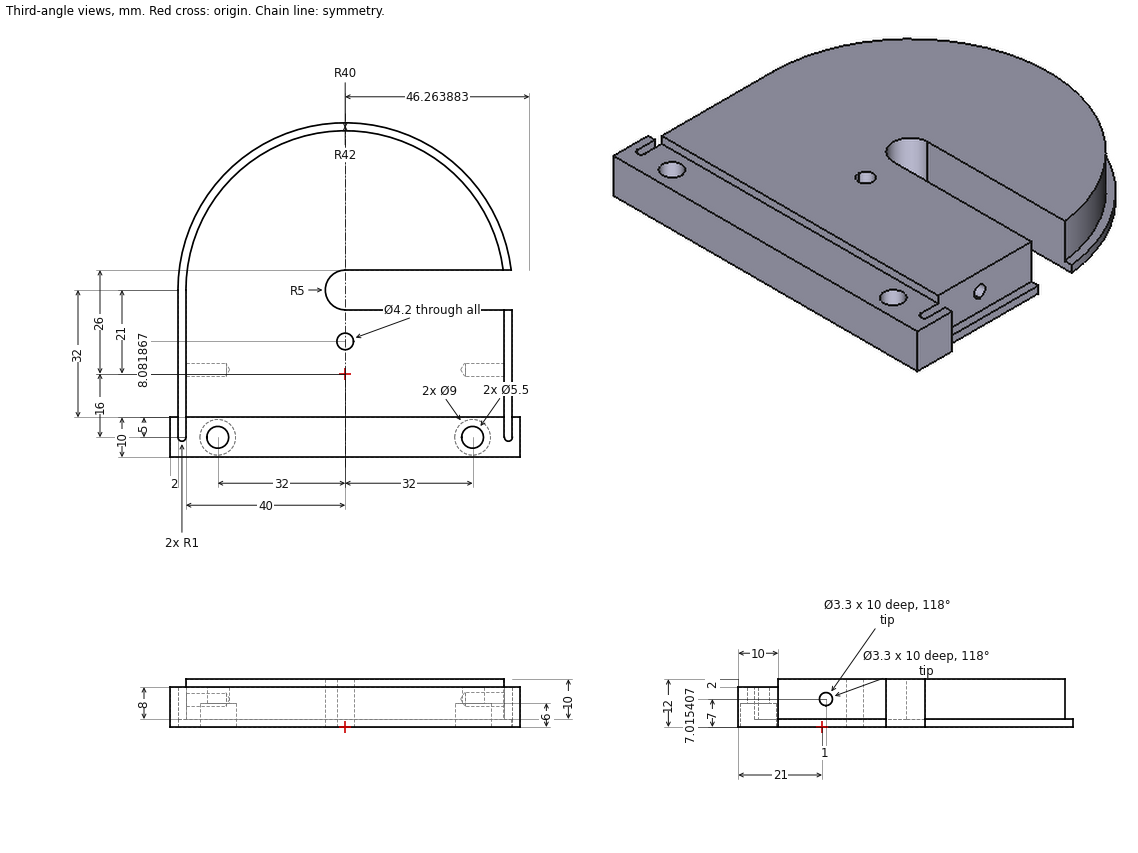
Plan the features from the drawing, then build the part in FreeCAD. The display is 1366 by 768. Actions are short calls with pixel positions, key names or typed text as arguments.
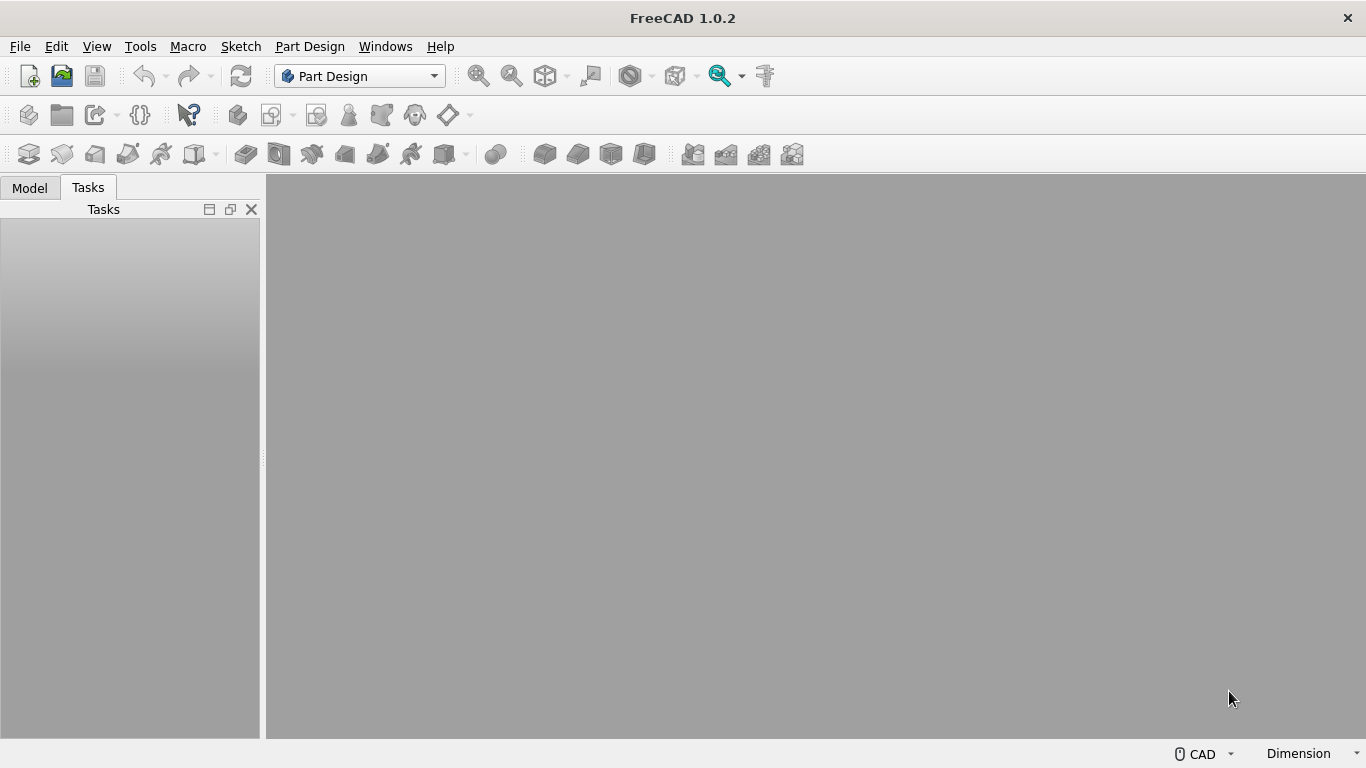
click(29, 76)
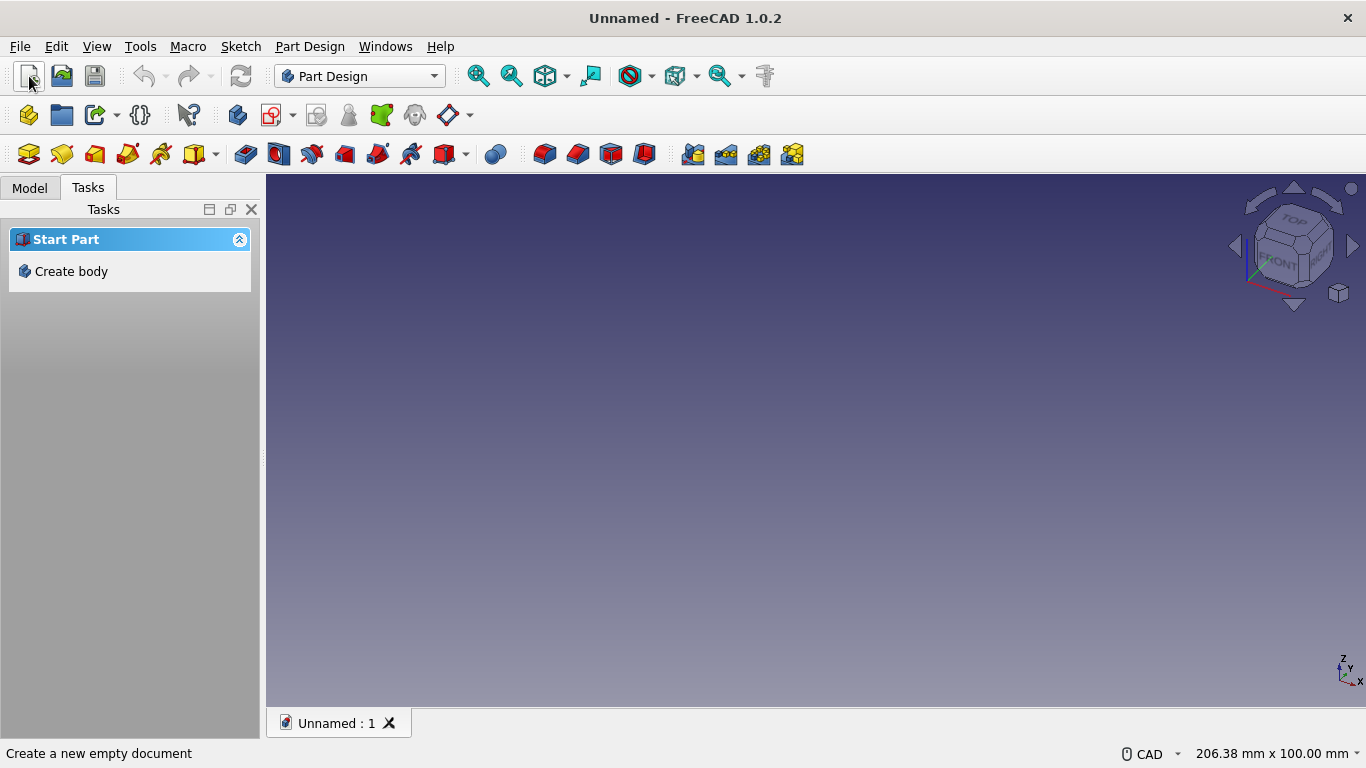
click(270, 116)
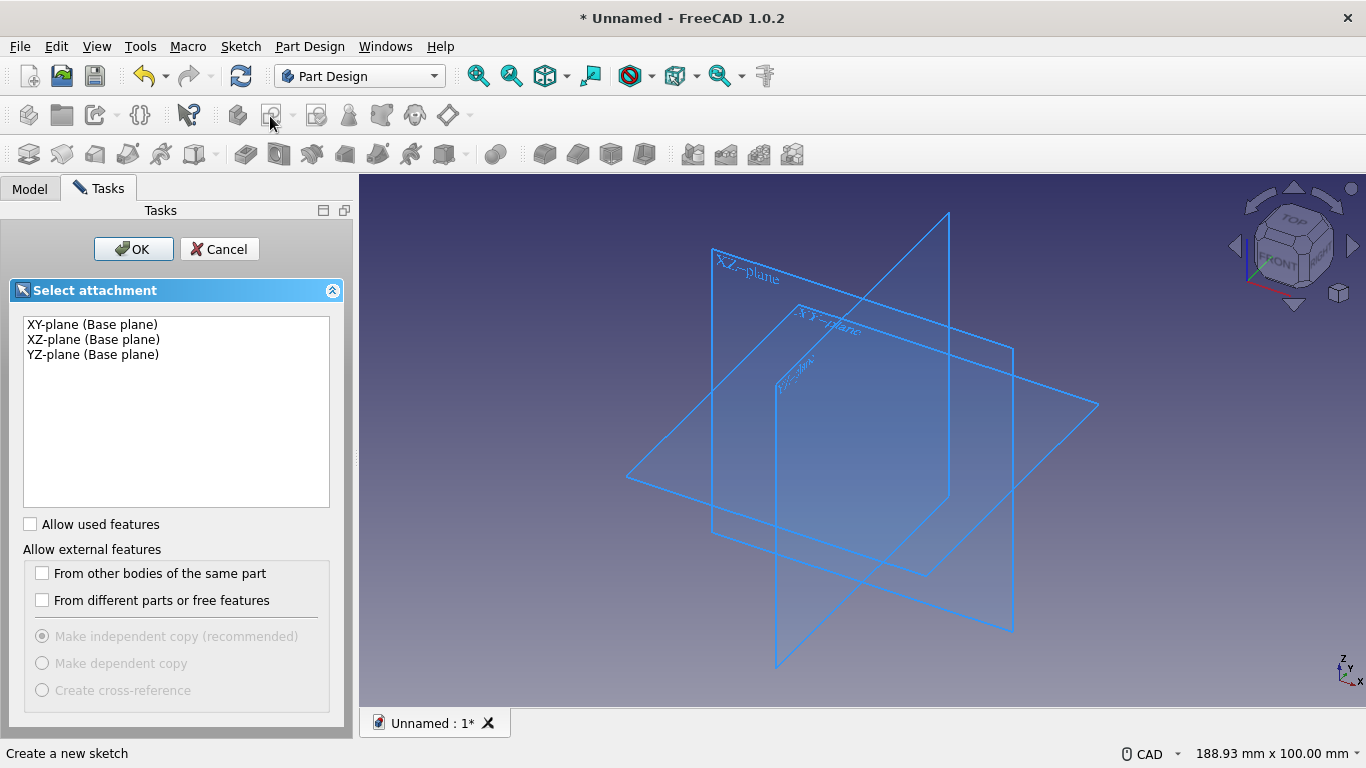
click(84, 324)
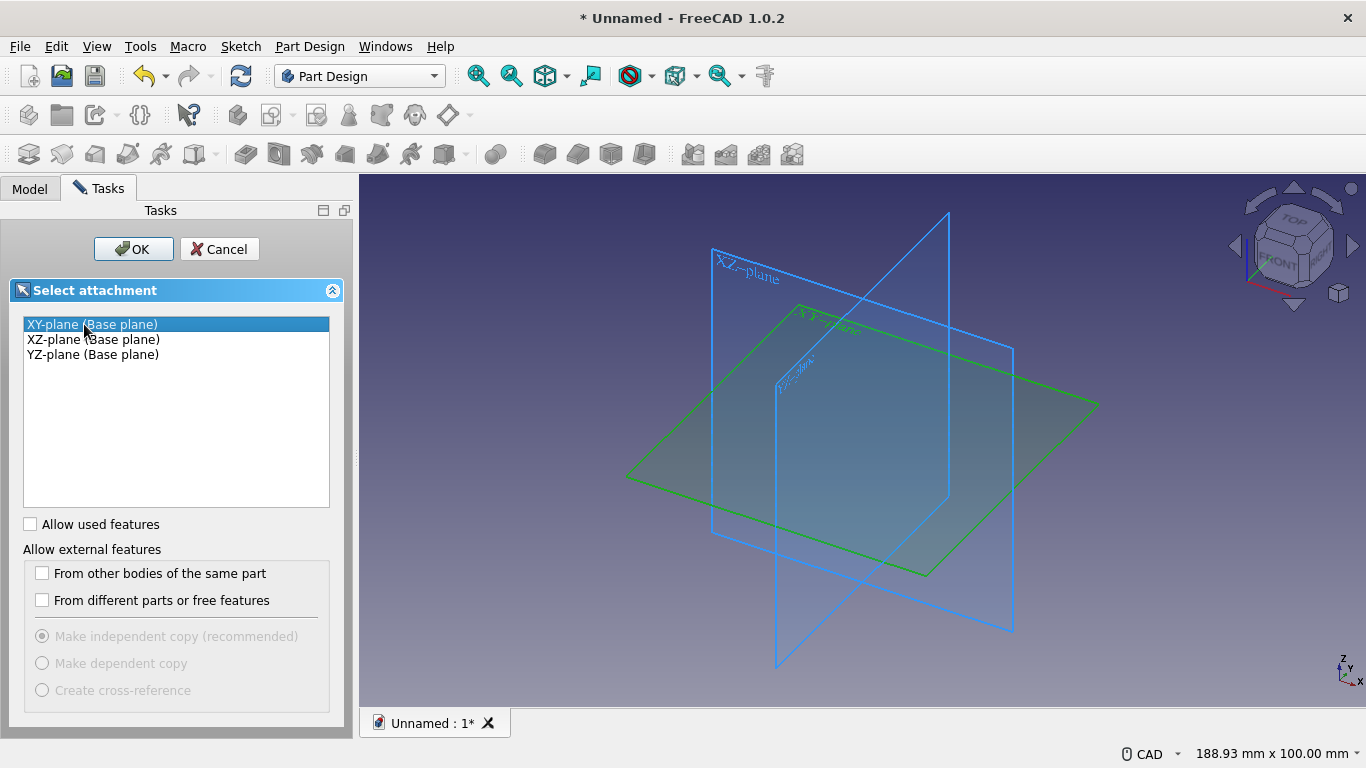
click(134, 249)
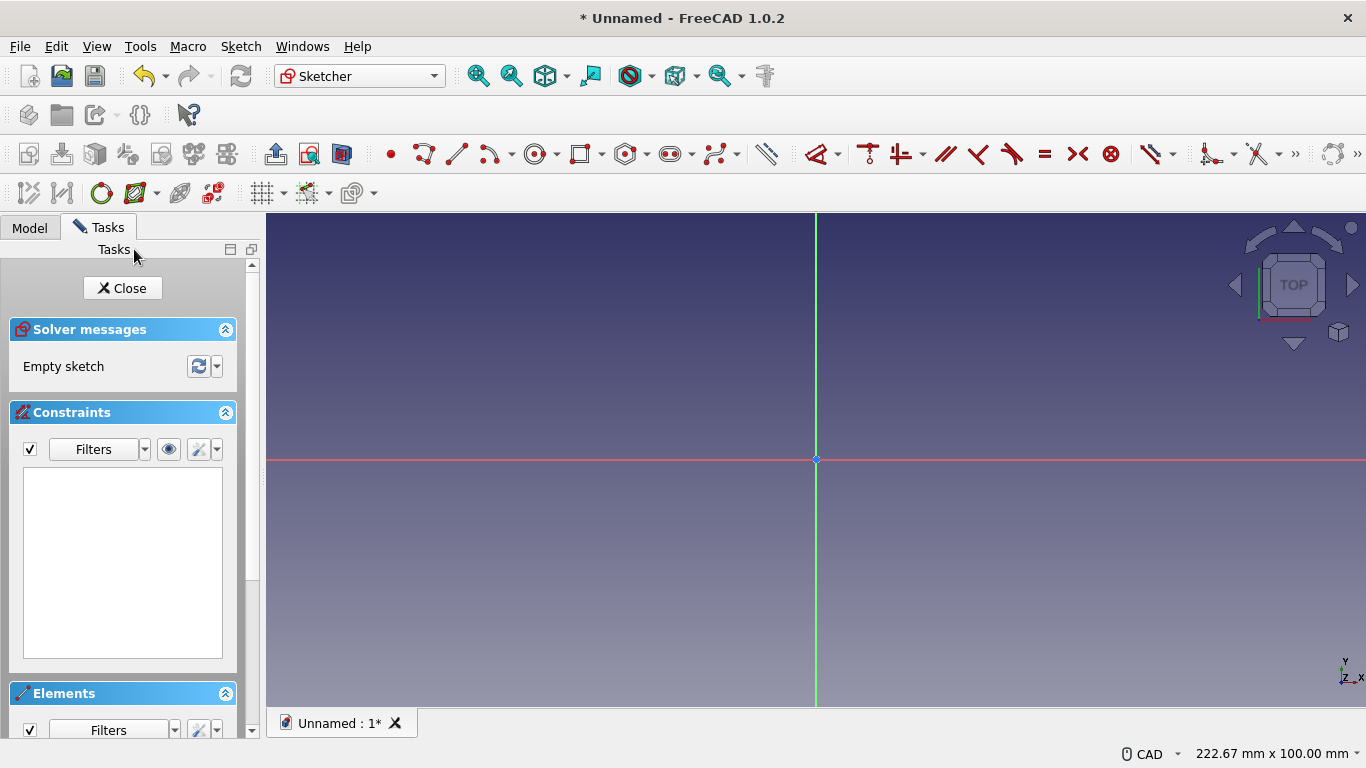
scroll(608, 671, down, 2)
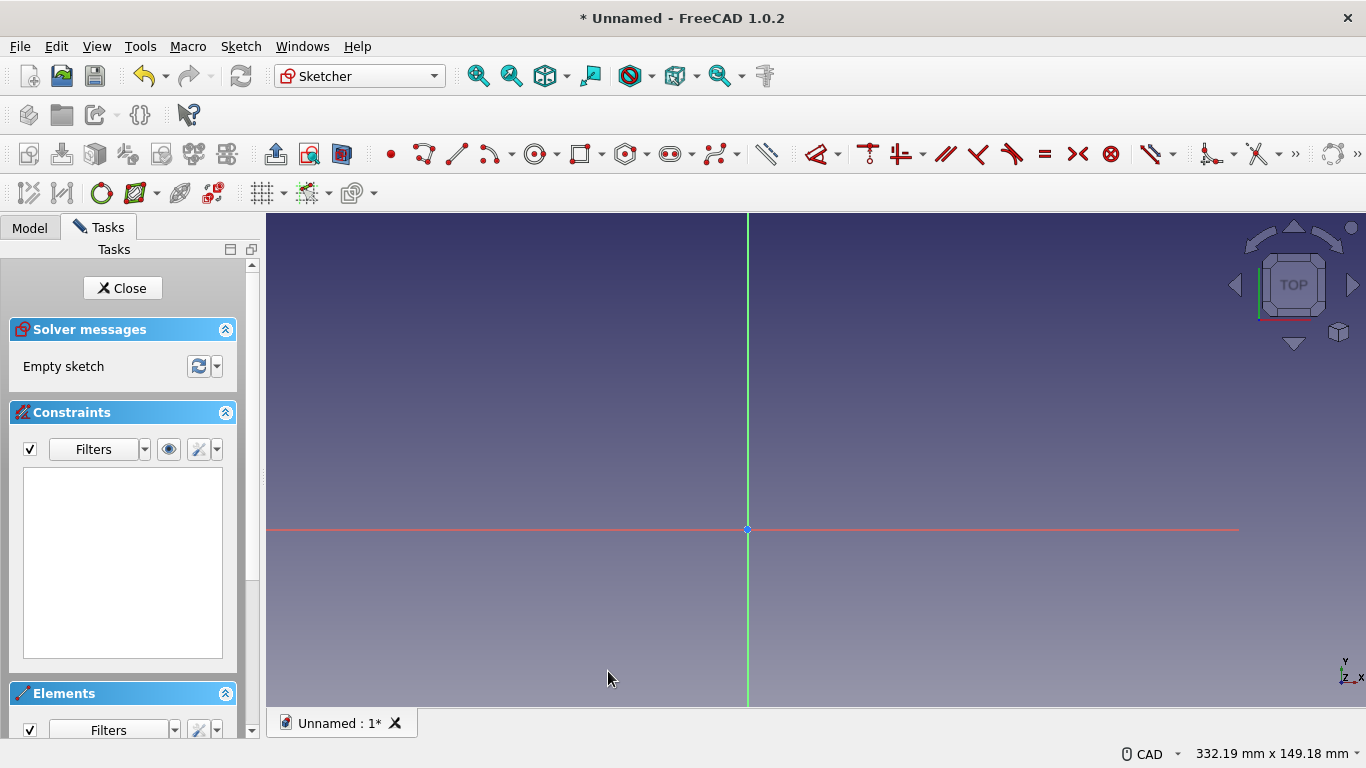
key(g)
key(m)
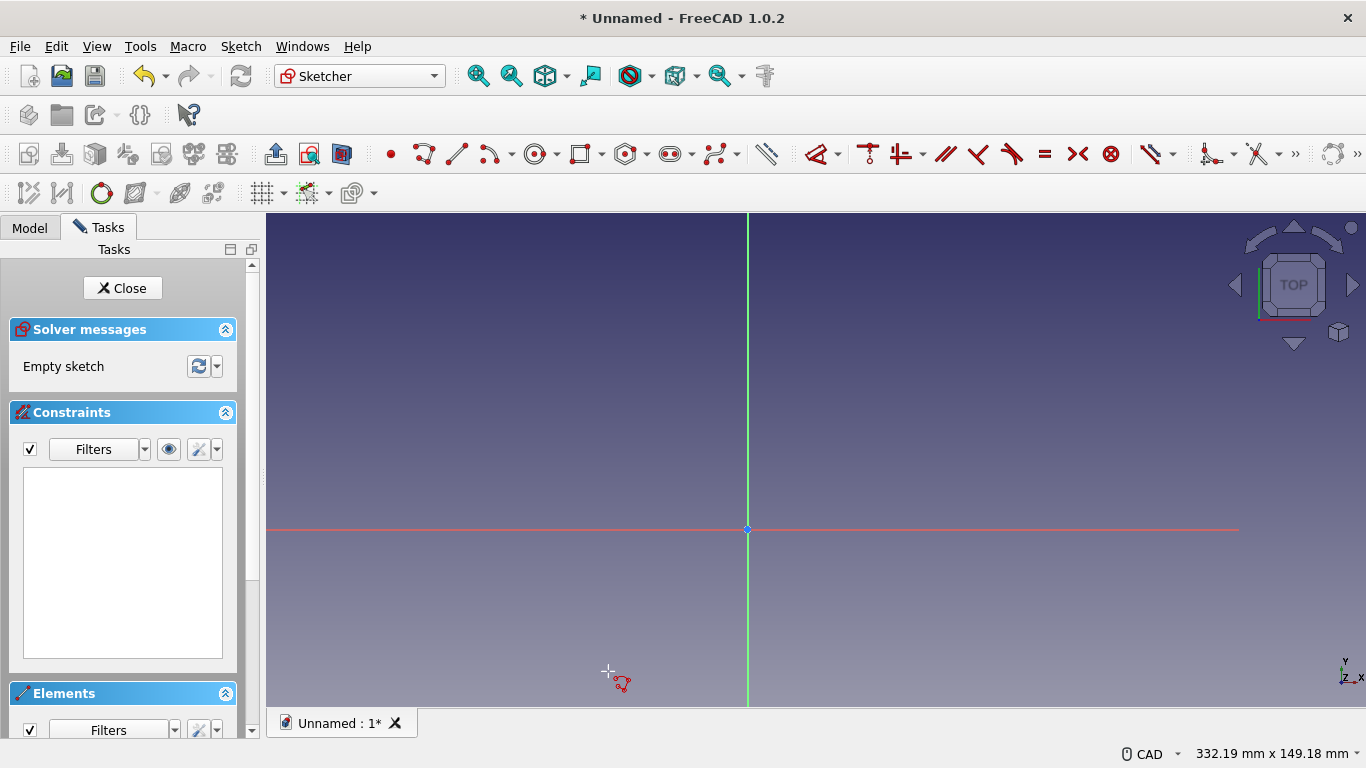
click(608, 460)
click(608, 566)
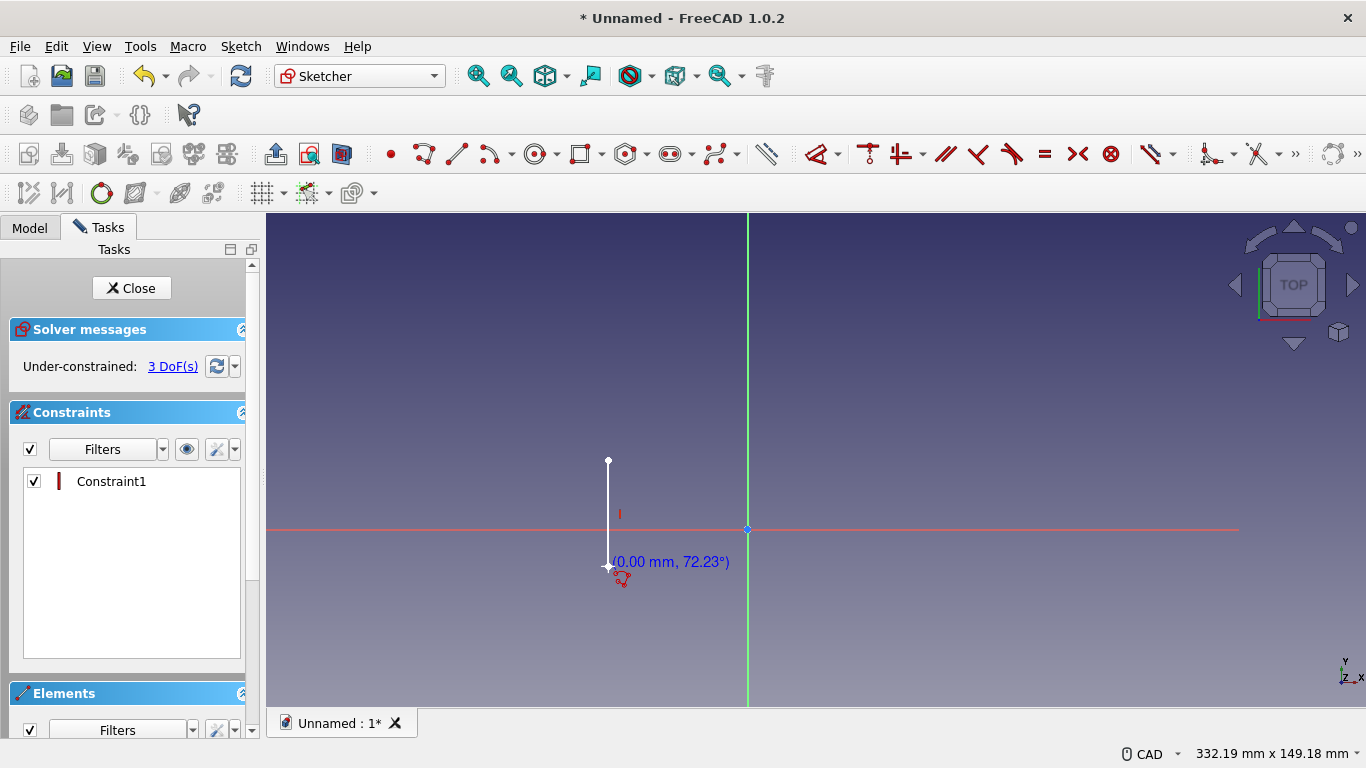
scroll(602, 566, up, 5)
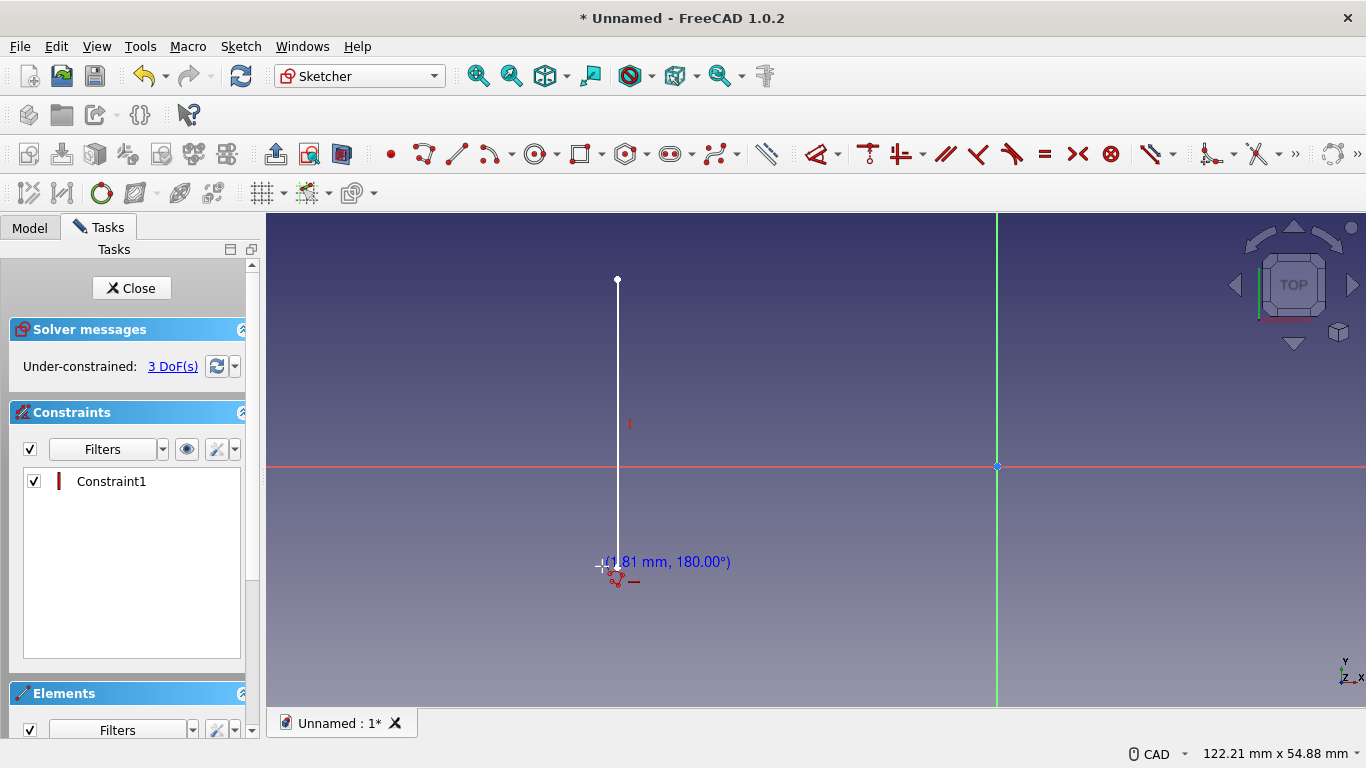
click(601, 565)
click(601, 656)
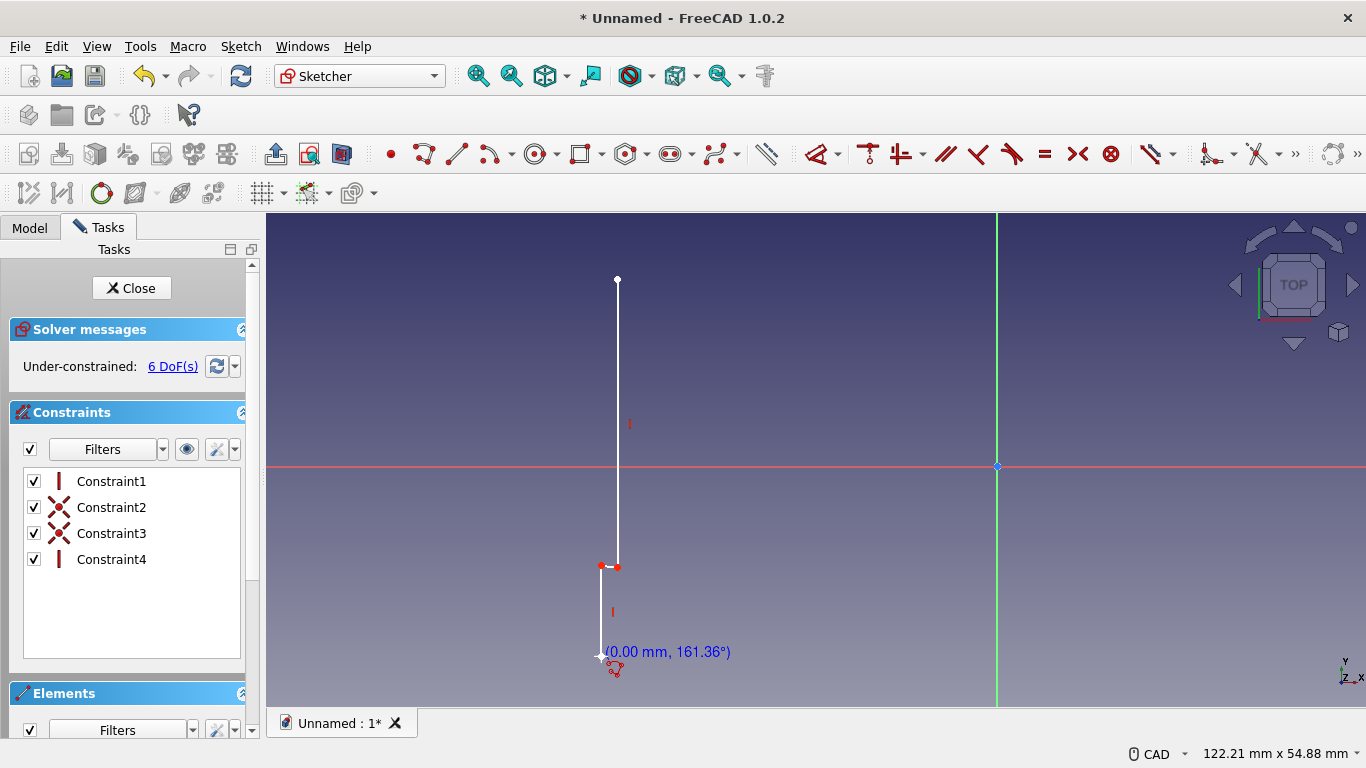
scroll(544, 609, down, 4)